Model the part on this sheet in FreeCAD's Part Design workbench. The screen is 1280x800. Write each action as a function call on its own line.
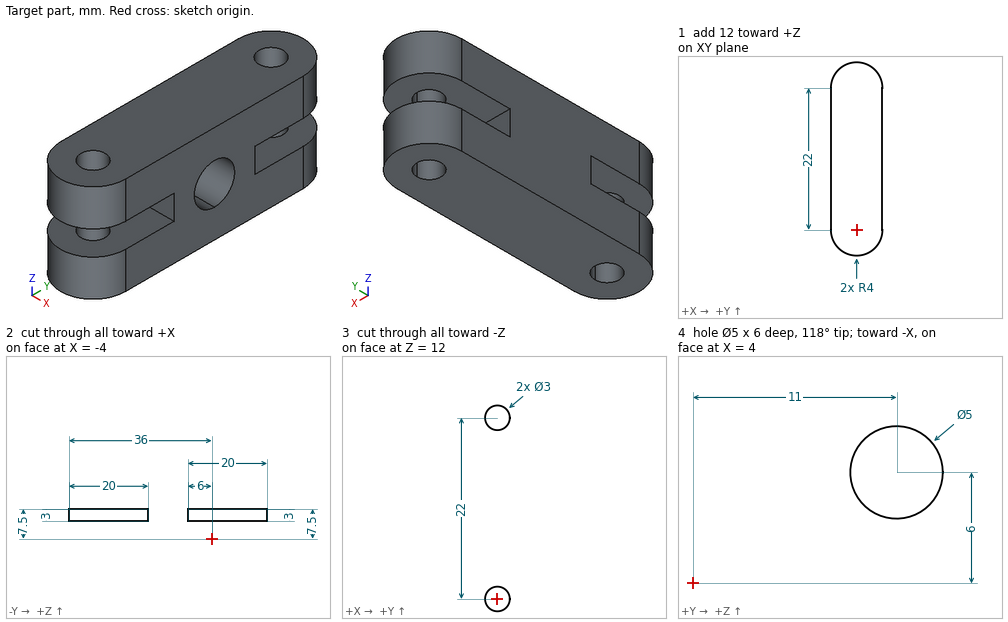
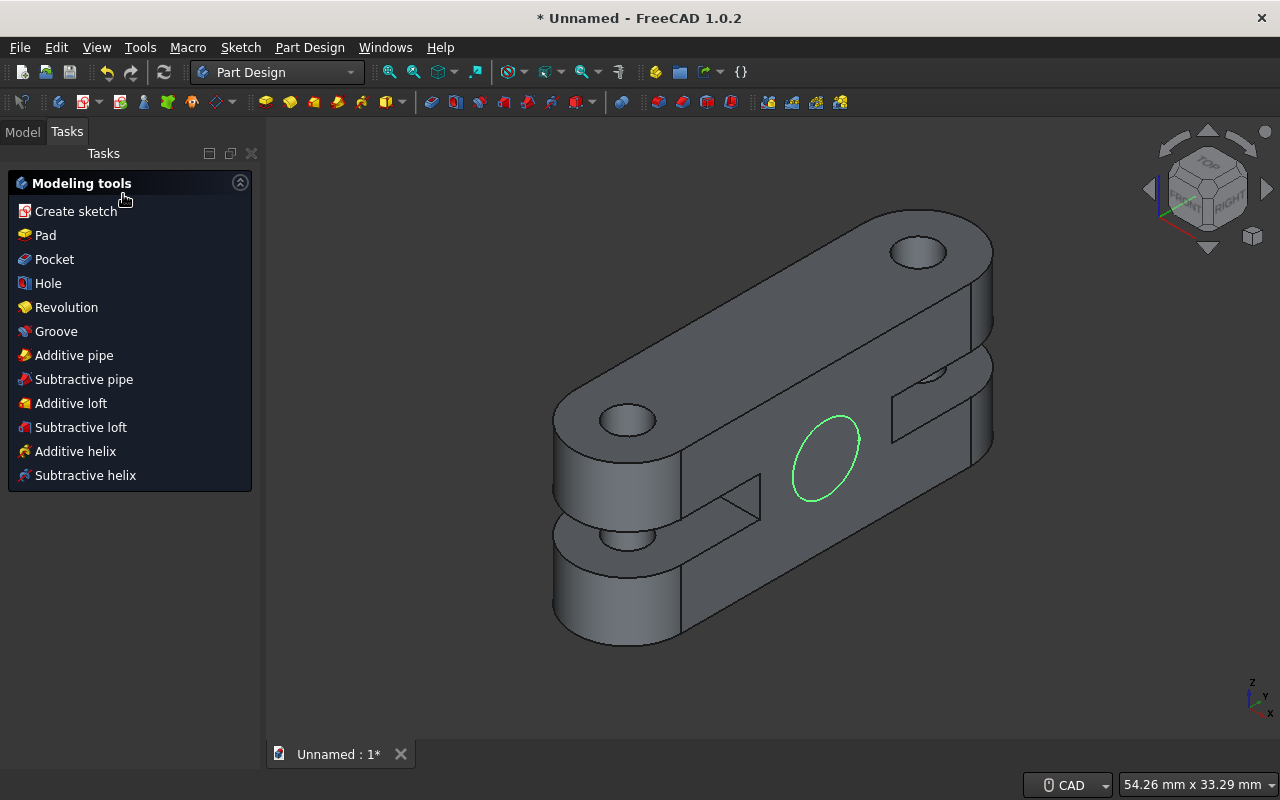
click(456, 102)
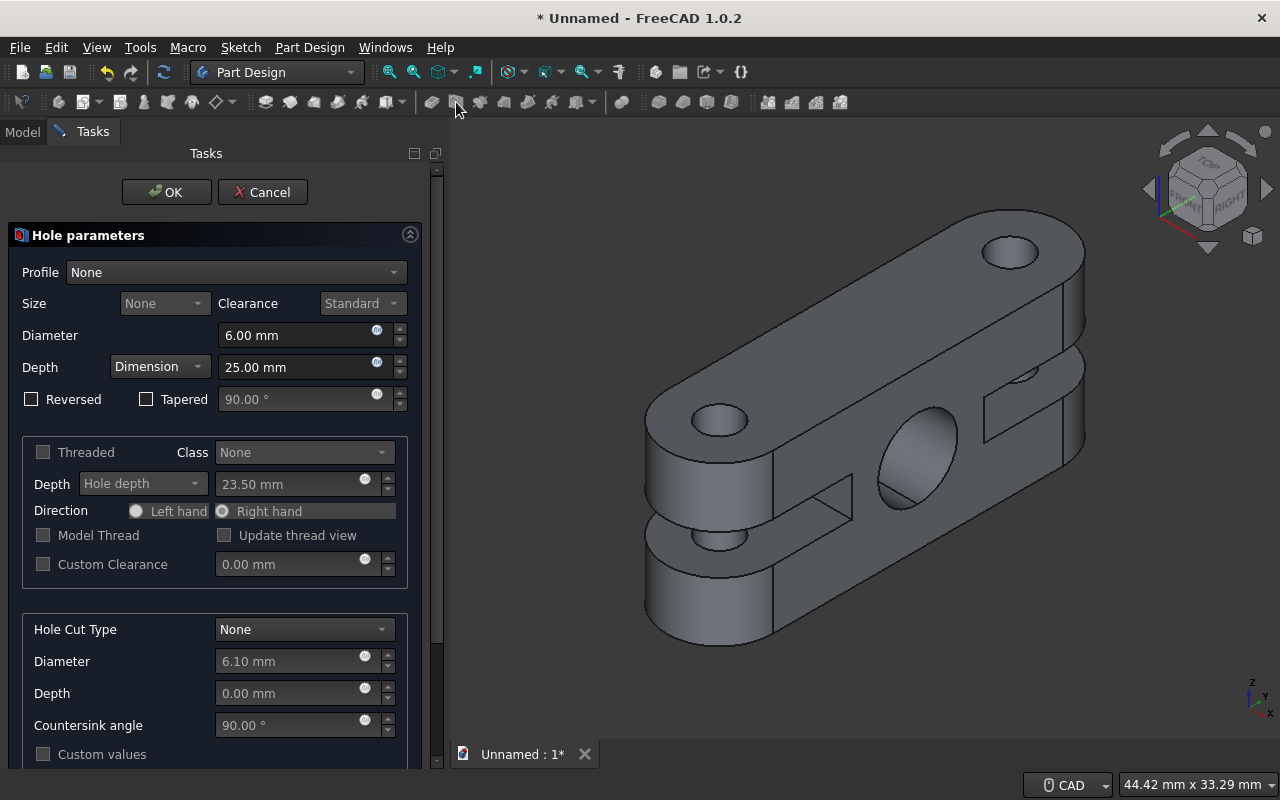
triple_click(305, 335)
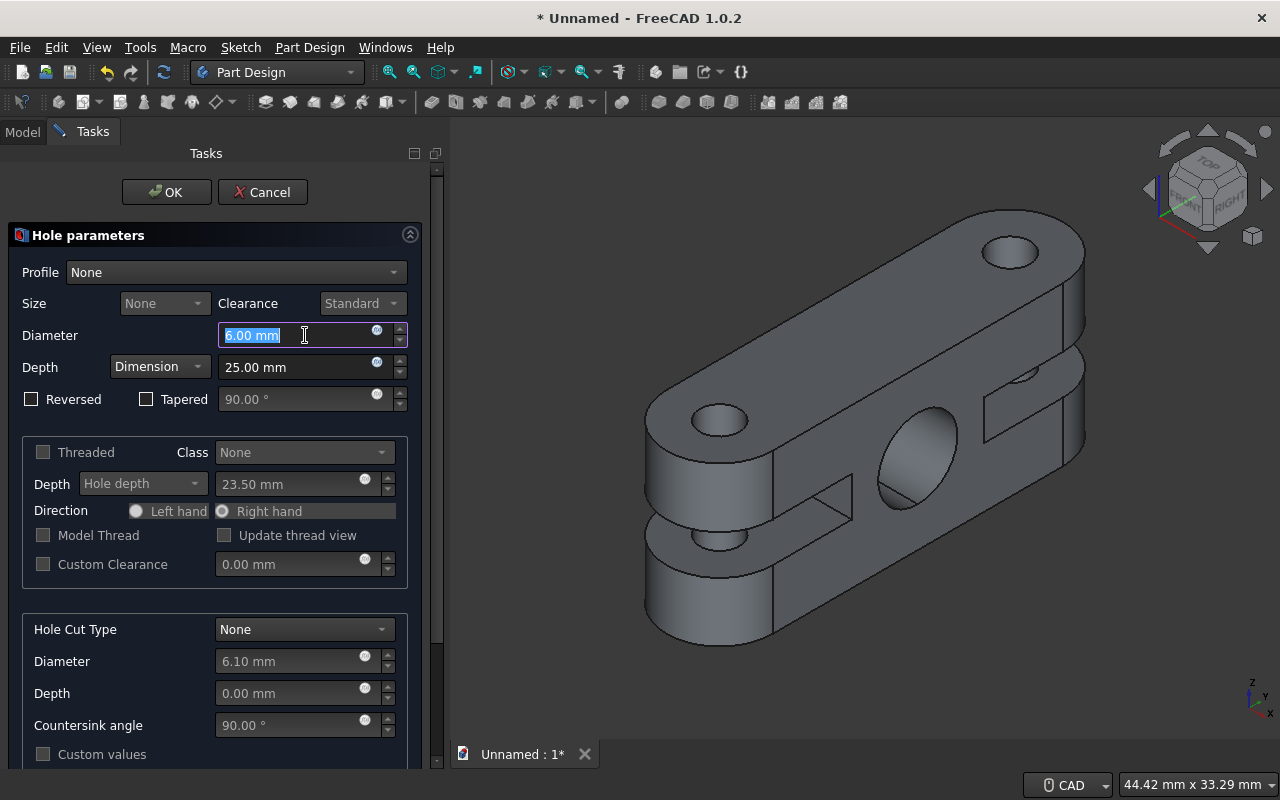
text(5)
key(Tab)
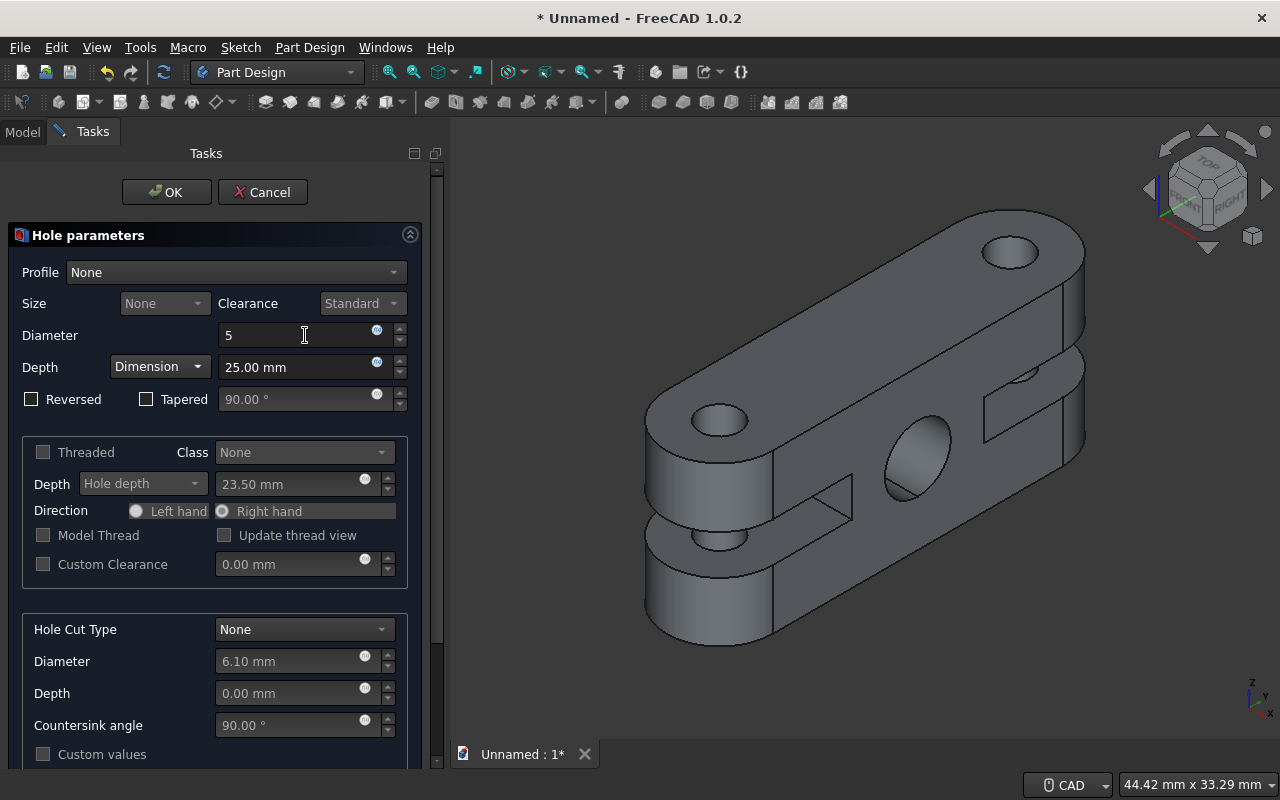
triple_click(305, 367)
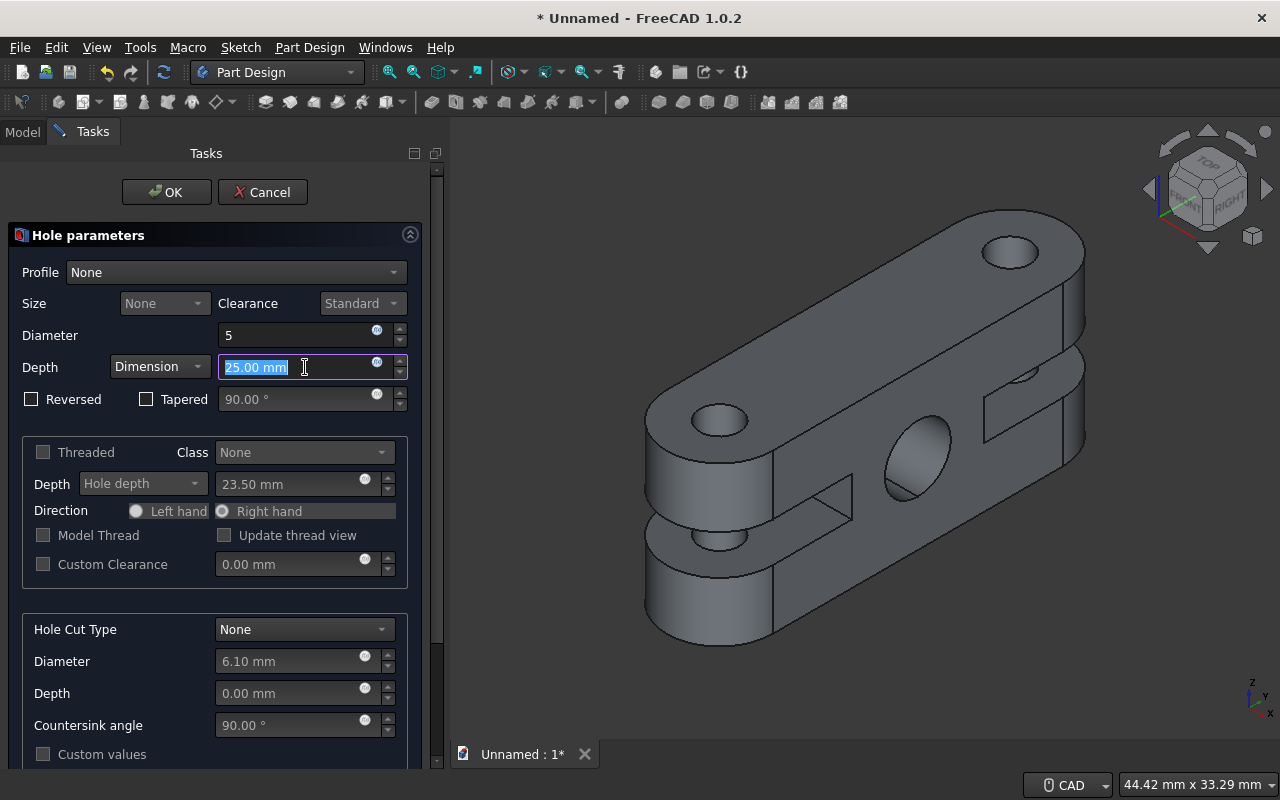
text(6)
key(Tab)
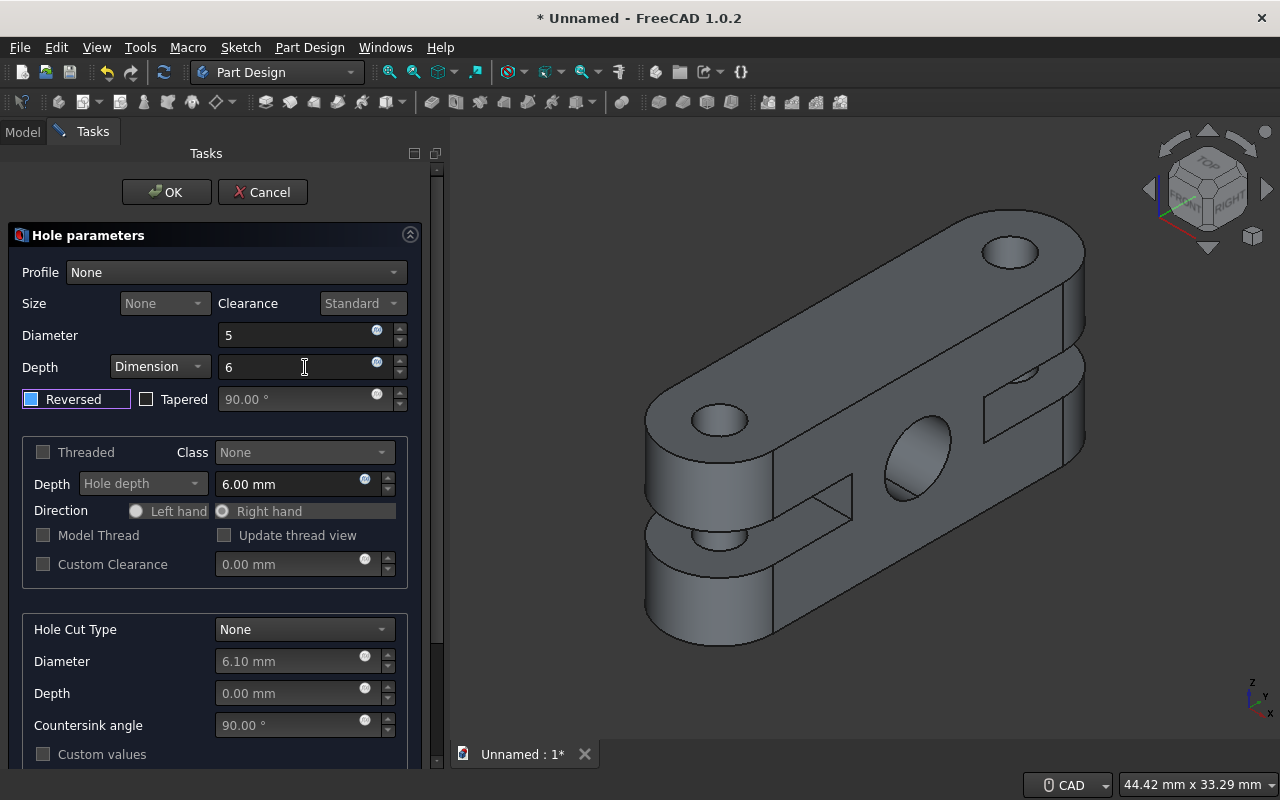
click(167, 192)